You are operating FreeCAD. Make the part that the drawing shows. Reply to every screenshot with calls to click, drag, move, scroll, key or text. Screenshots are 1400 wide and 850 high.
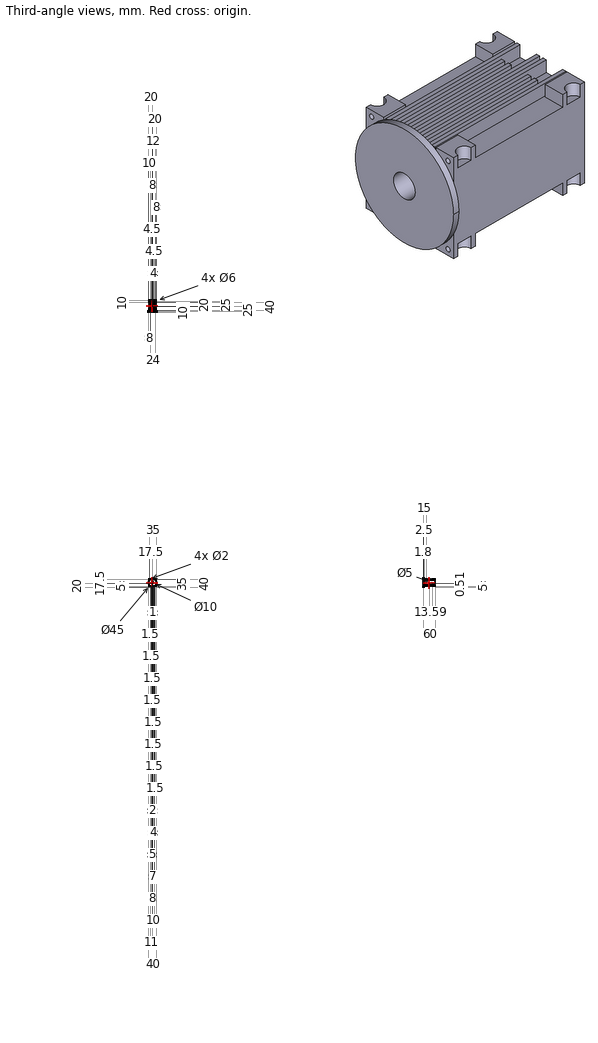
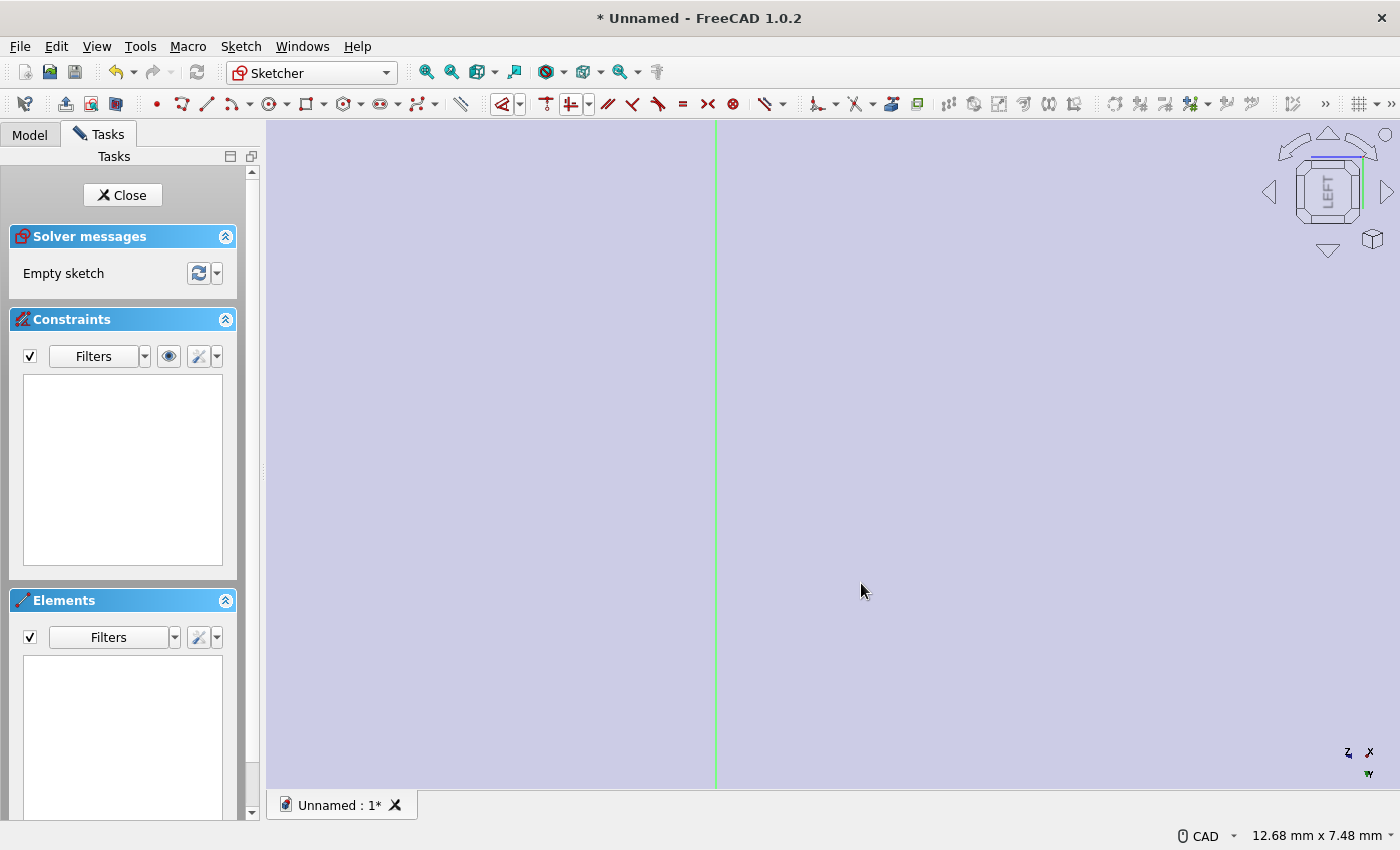
key(g)
key(c)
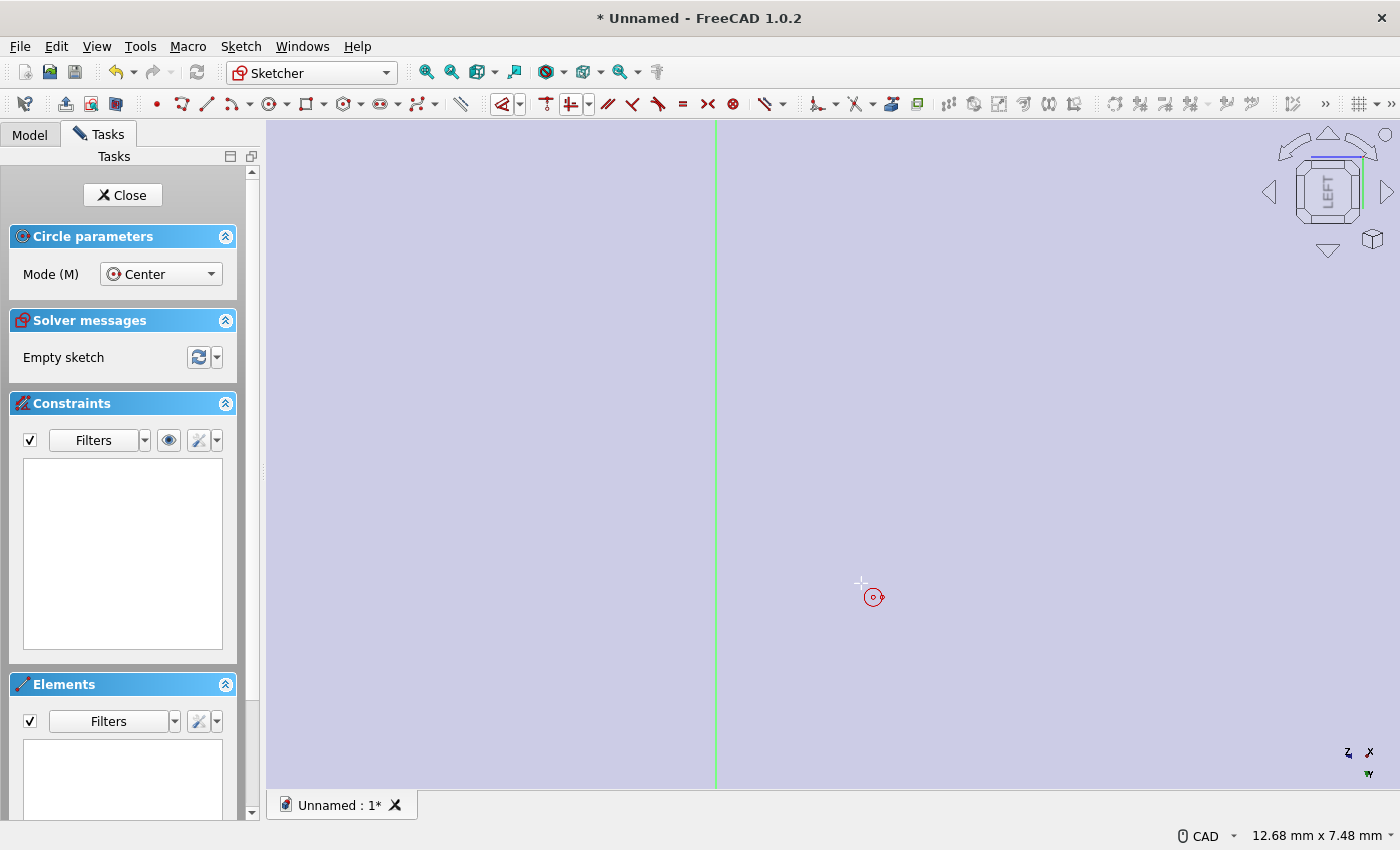
click(762, 443)
click(920, 285)
key(Escape)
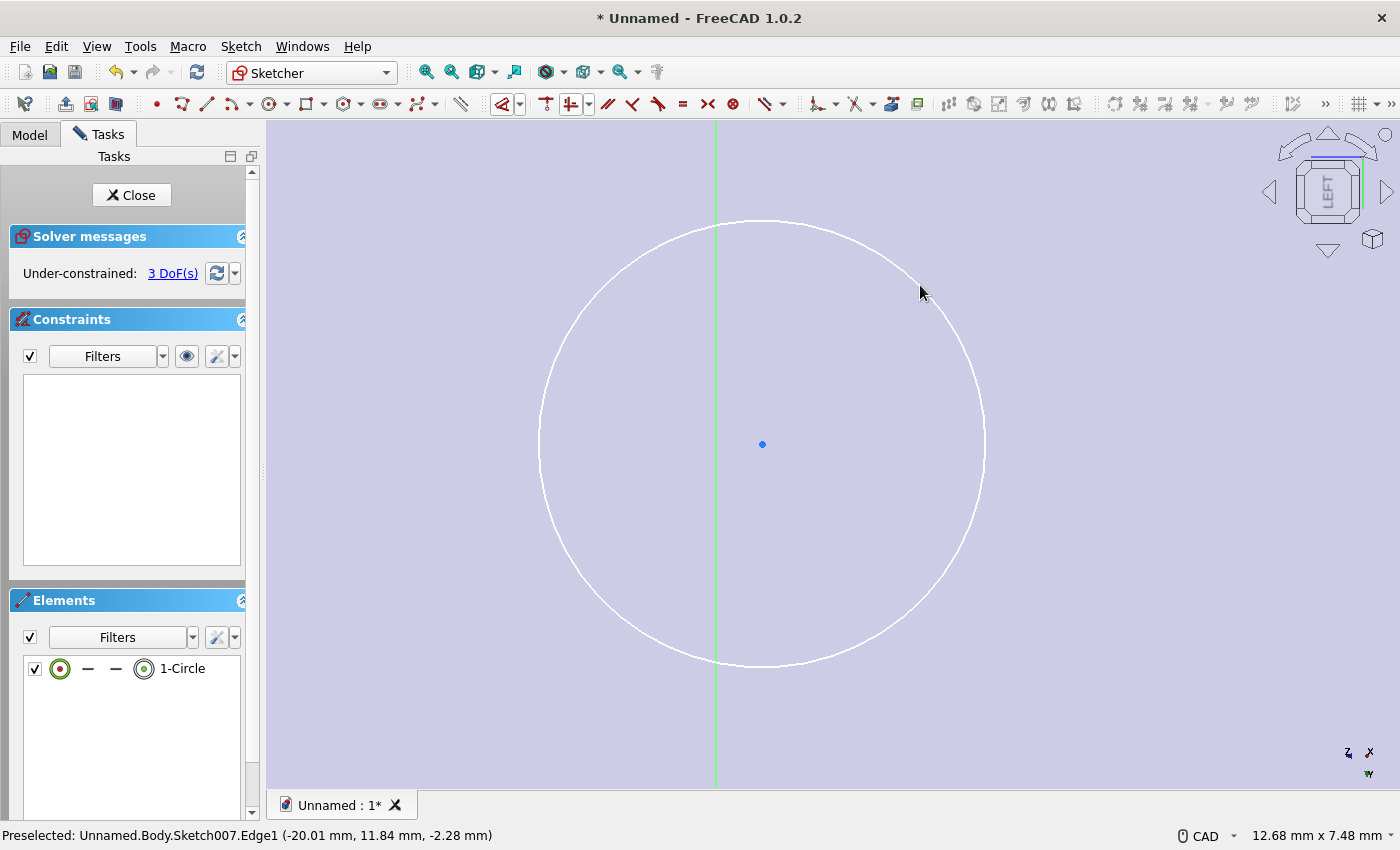
click(920, 286)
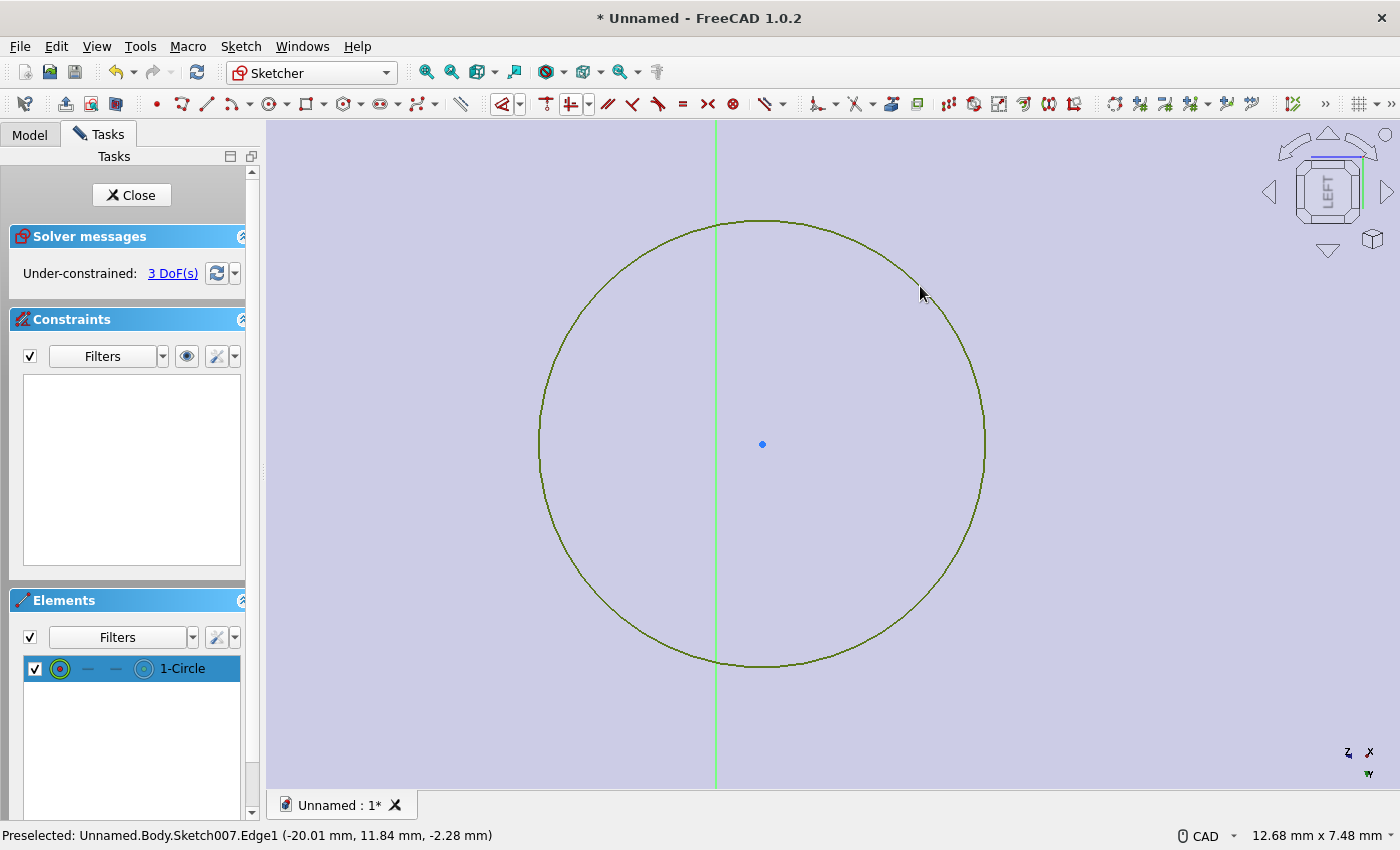
click(520, 104)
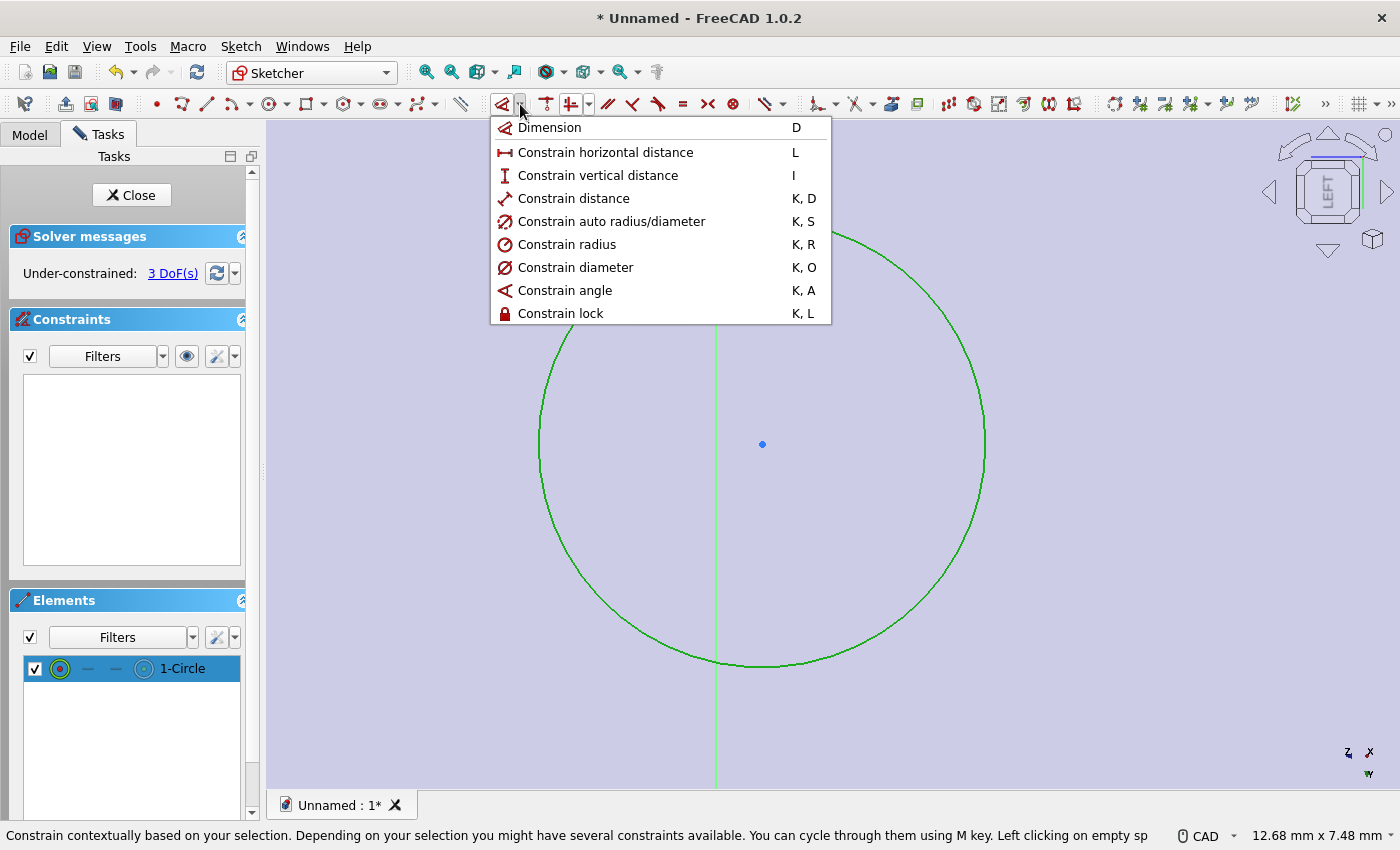
click(661, 268)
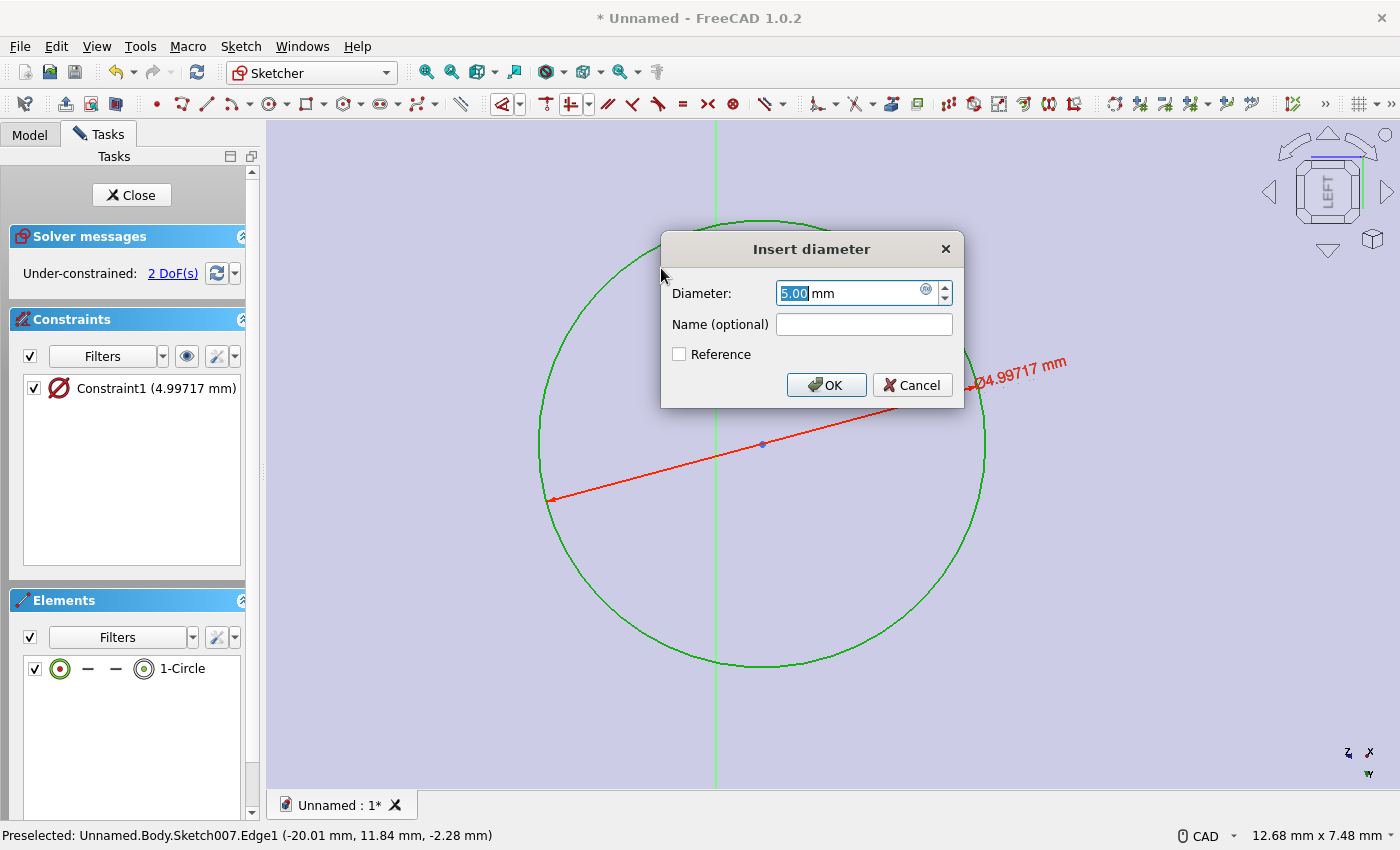
text(5)
key(Return)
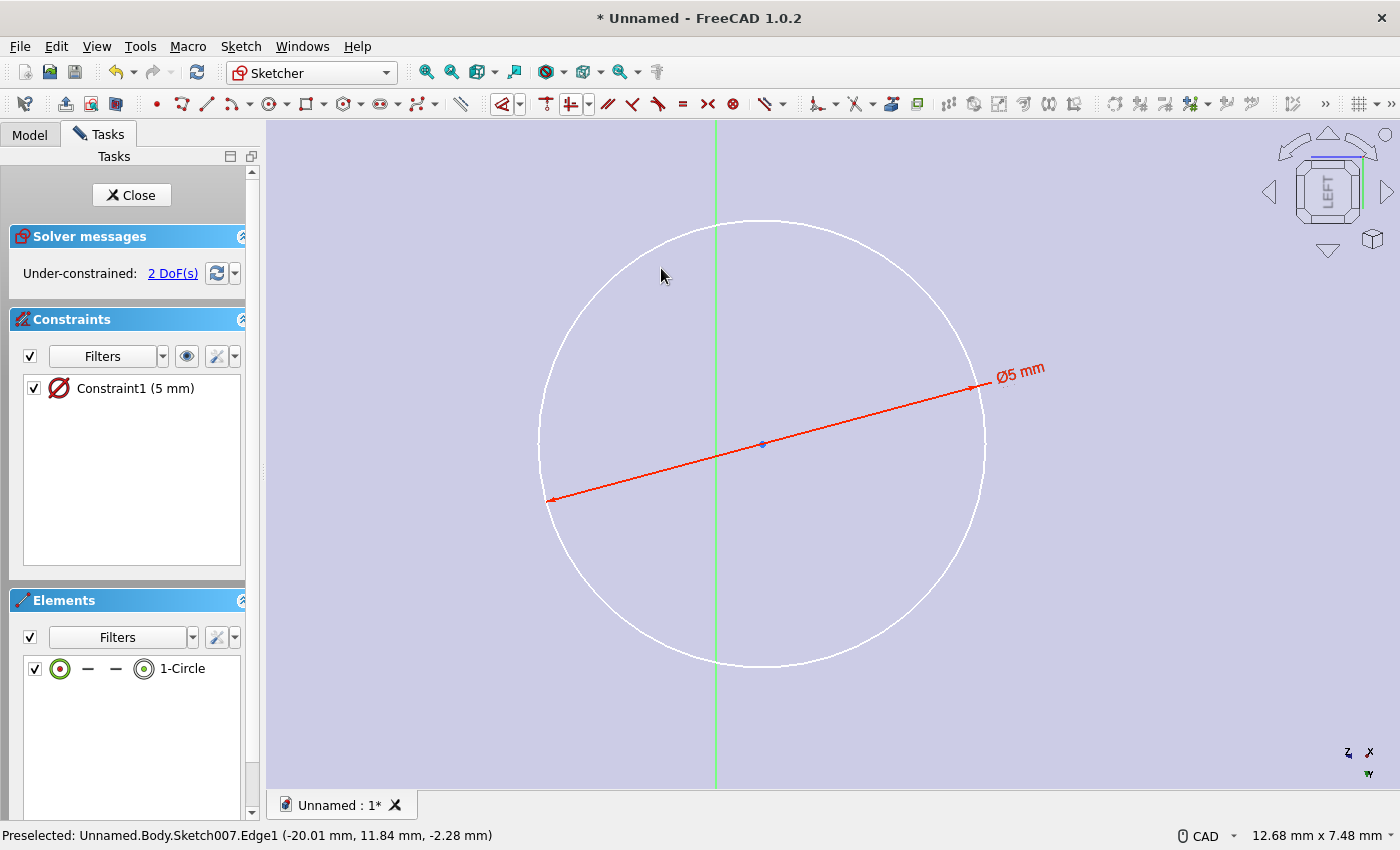
click(762, 444)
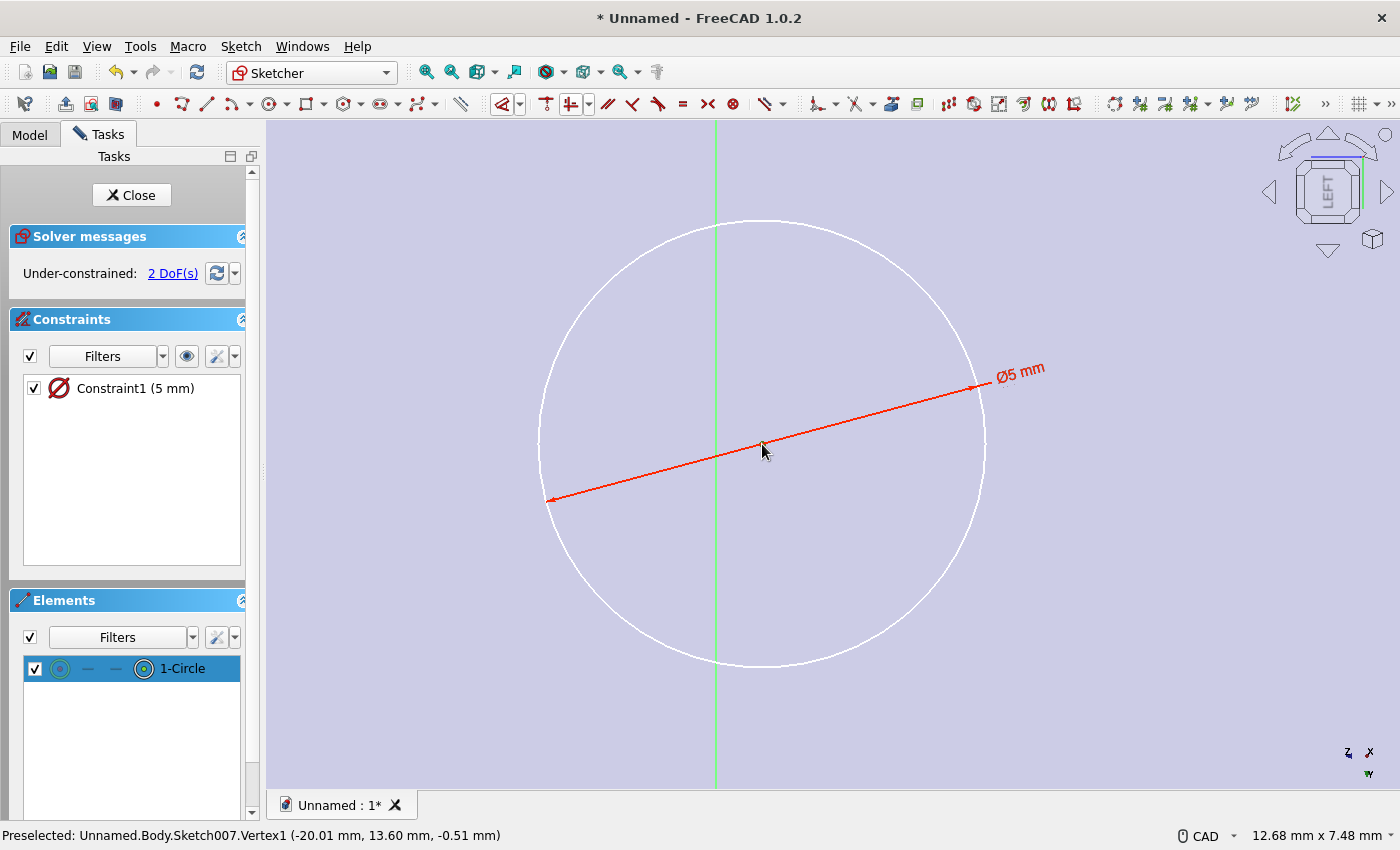
click(520, 104)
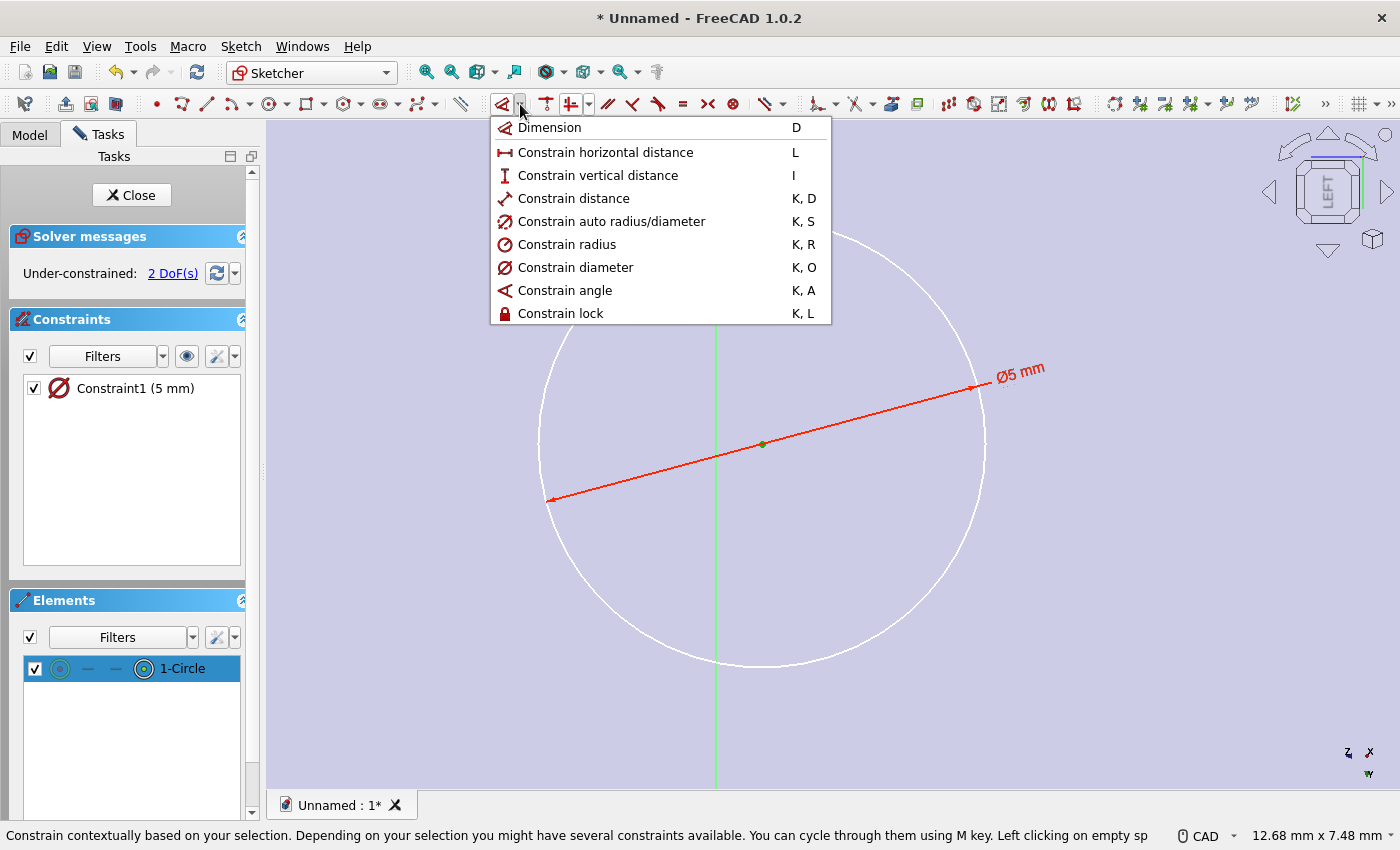
click(661, 152)